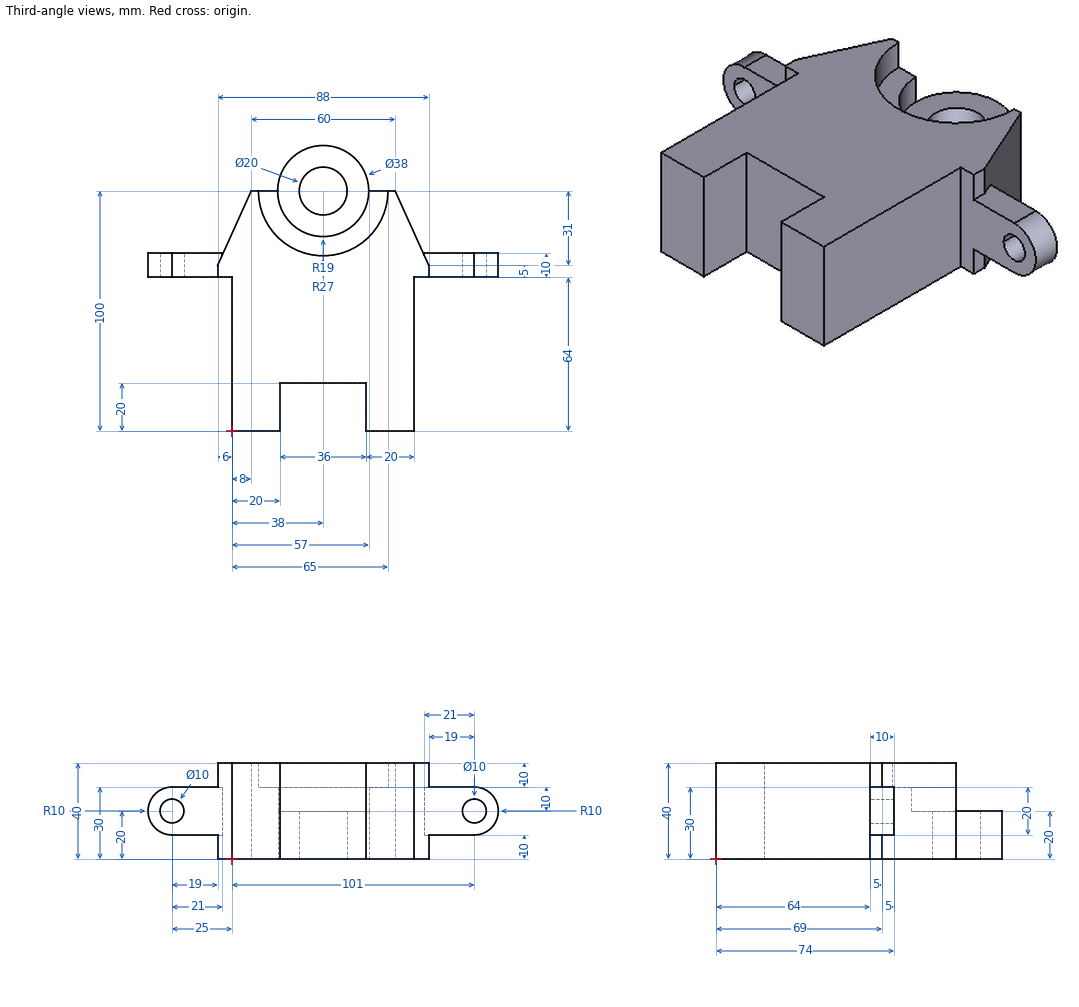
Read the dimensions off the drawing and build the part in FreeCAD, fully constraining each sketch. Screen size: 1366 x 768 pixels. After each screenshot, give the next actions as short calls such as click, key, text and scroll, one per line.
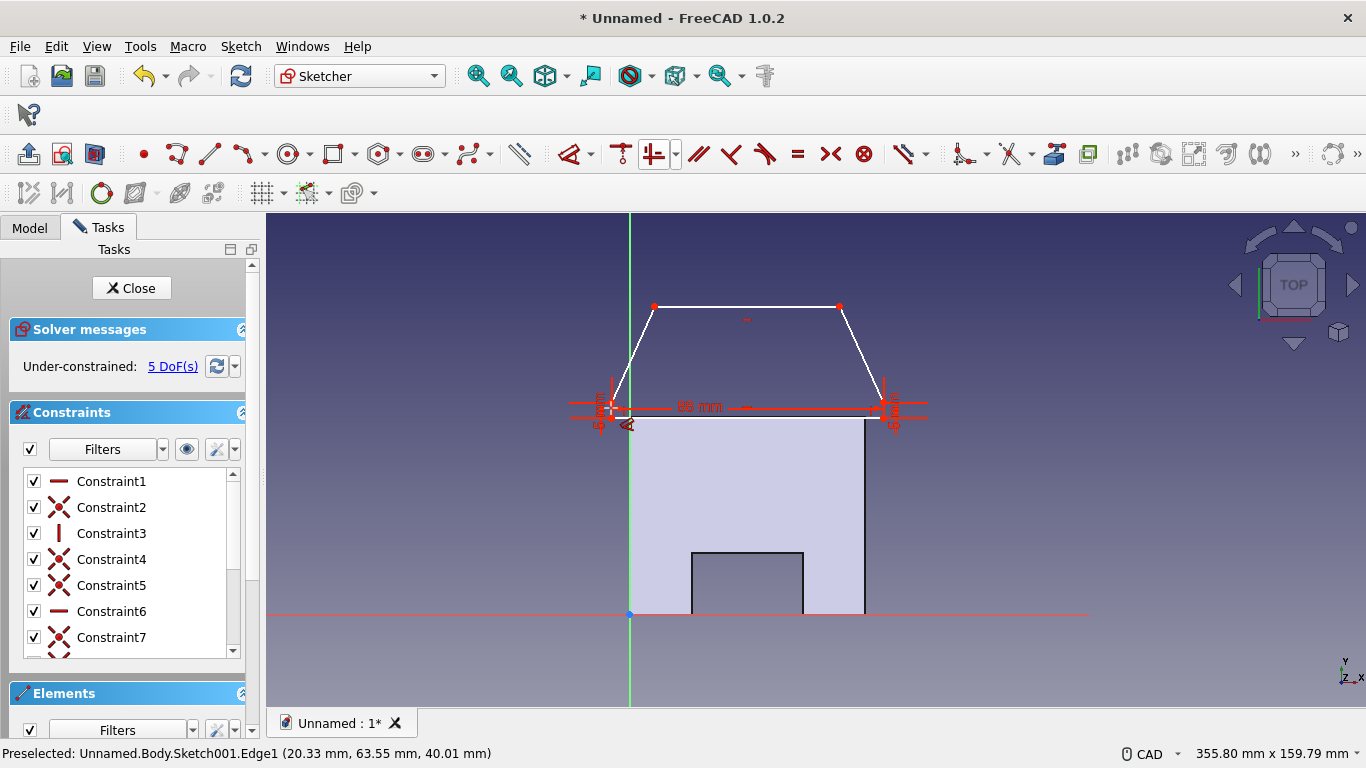
click(784, 307)
click(747, 273)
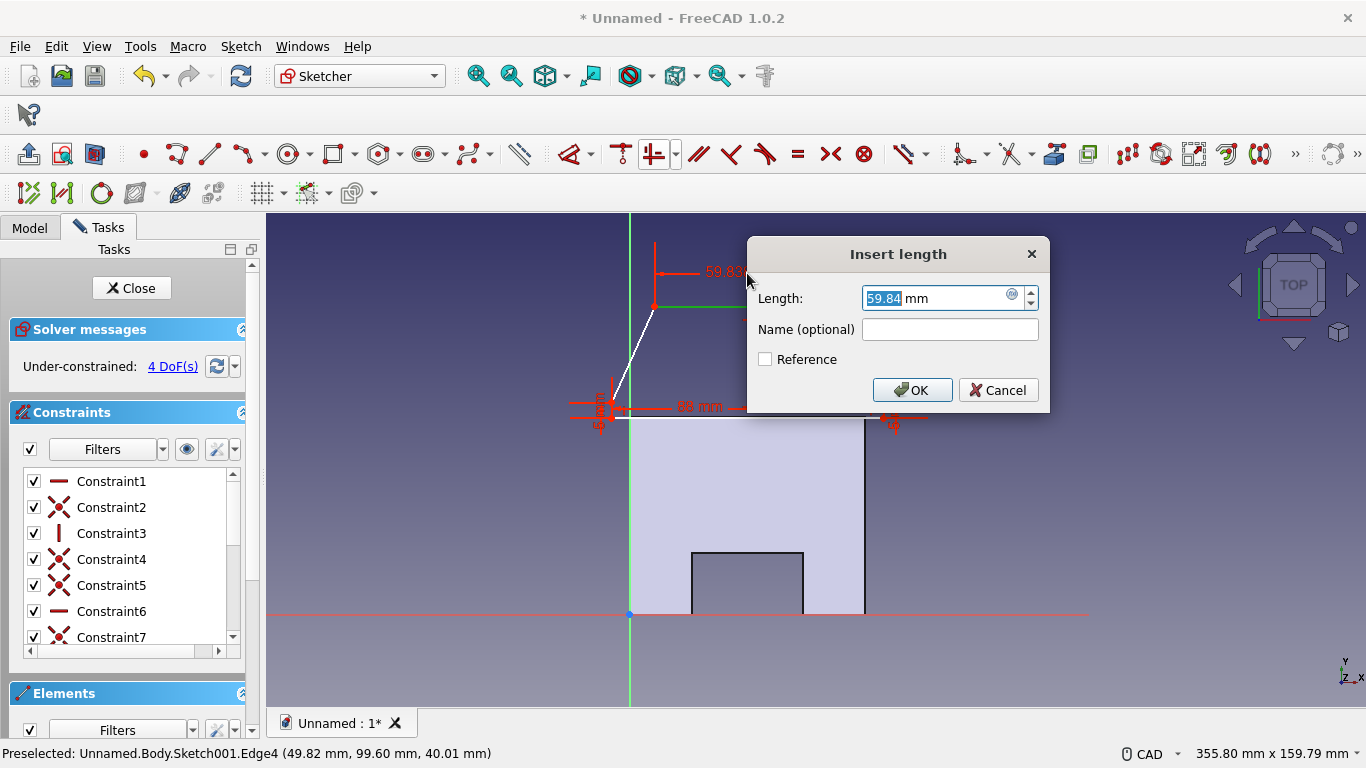
text(60)
key(Return)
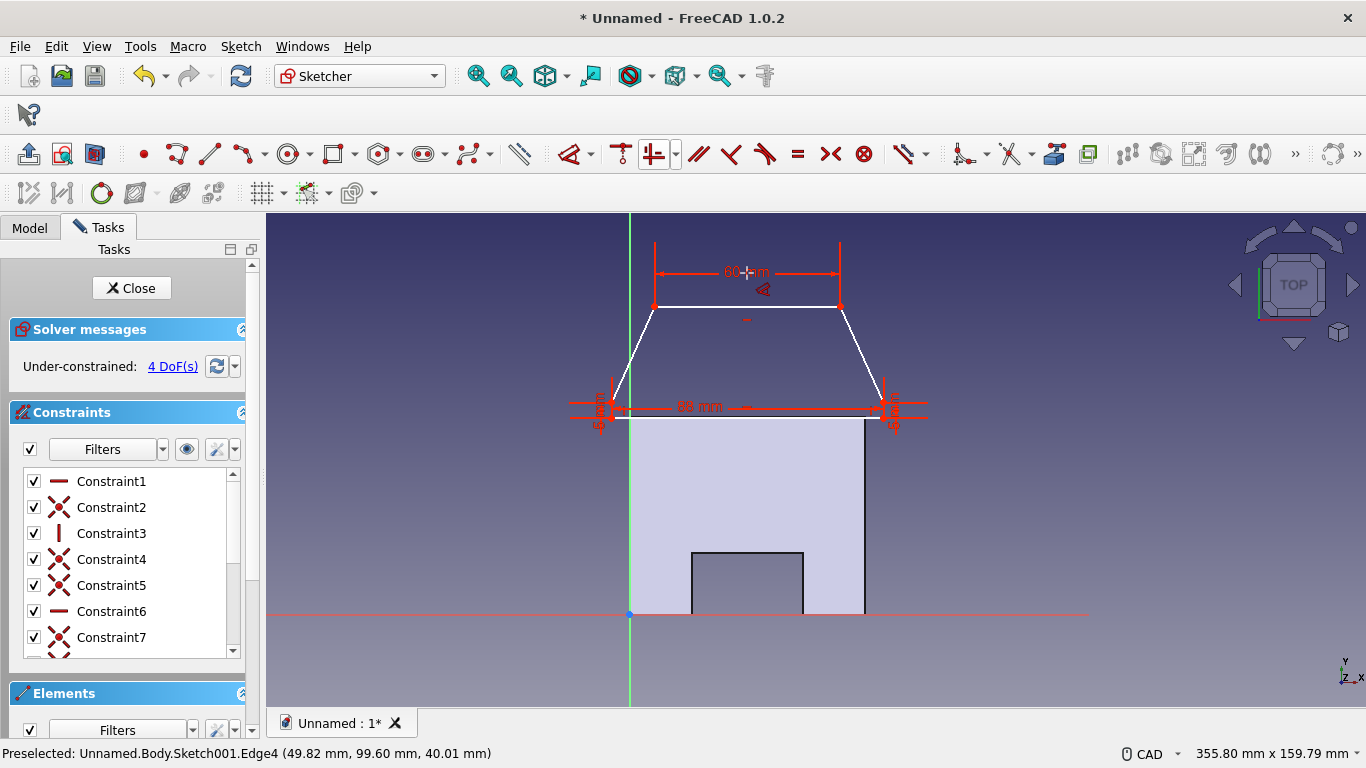
scroll(612, 418, up, 4)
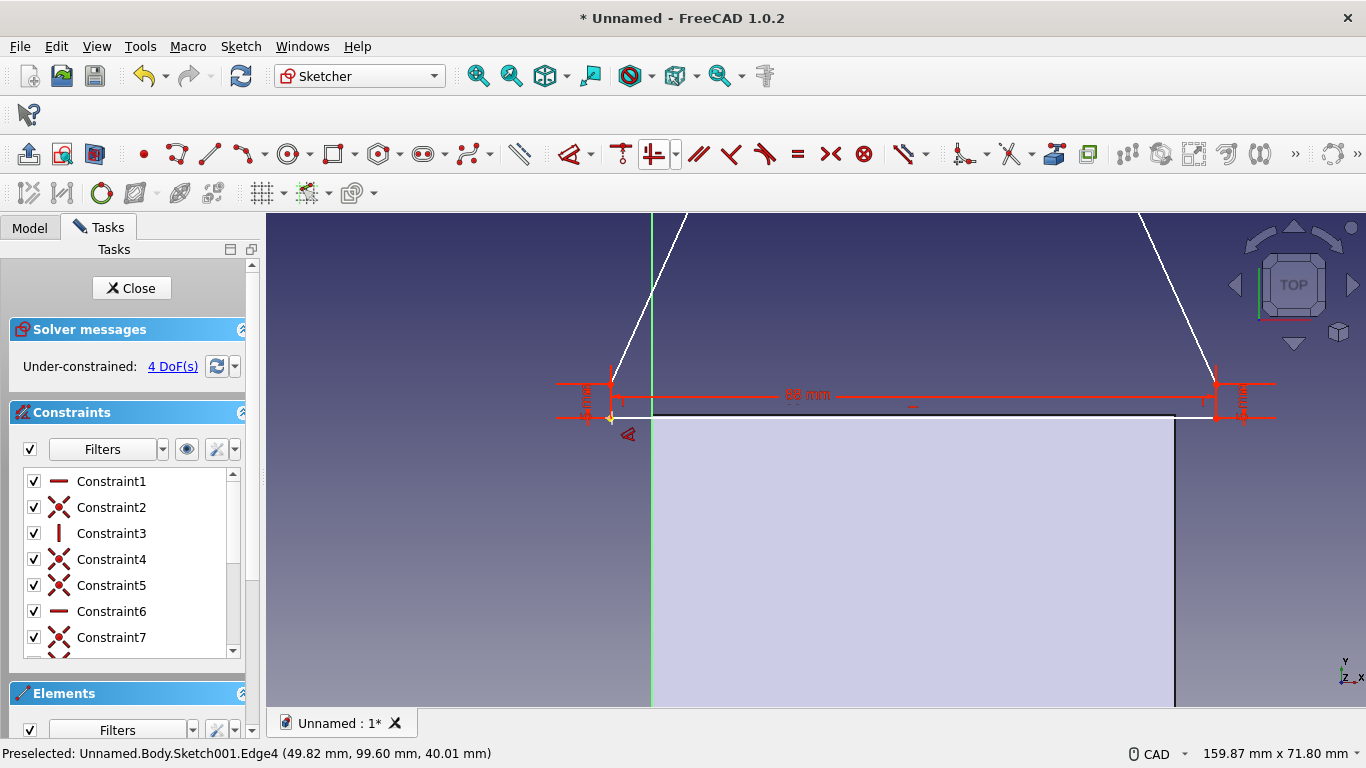
click(611, 418)
click(617, 336)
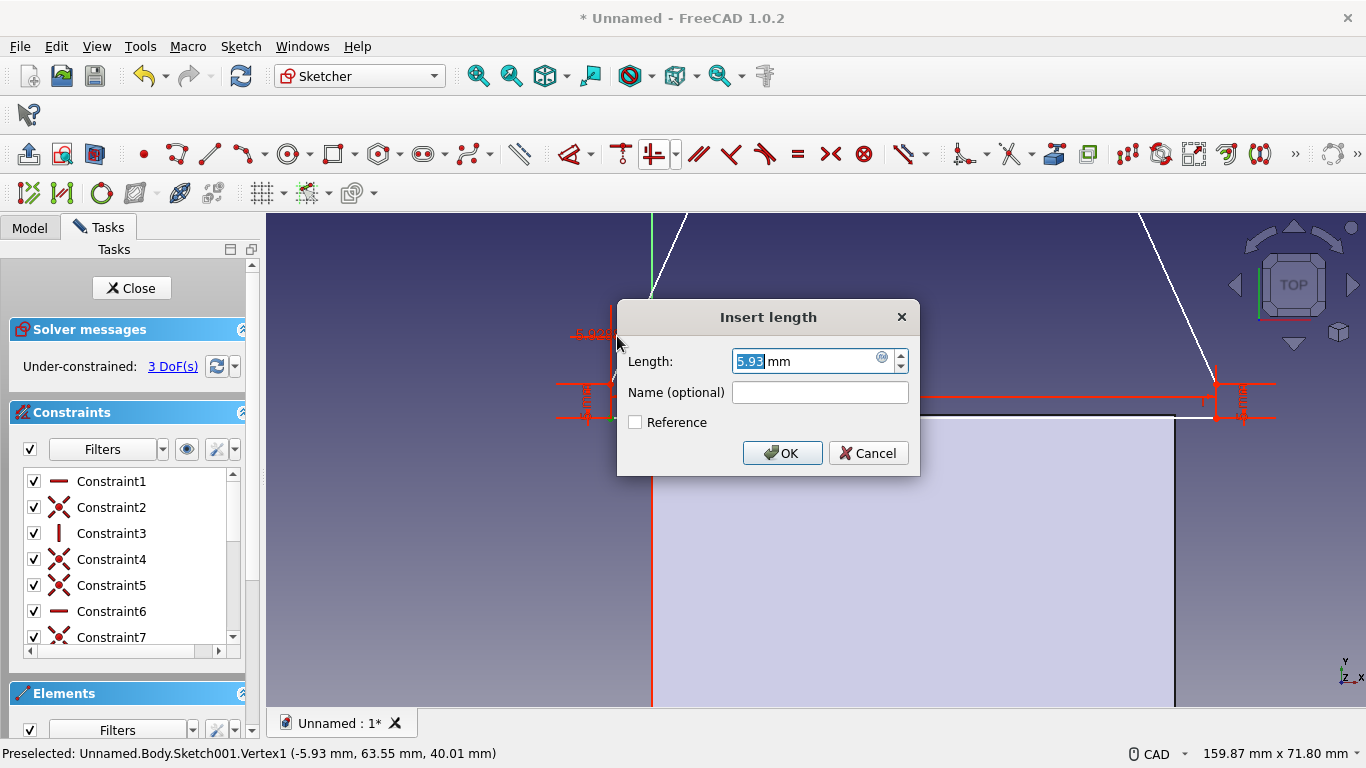
text(6)
key(Return)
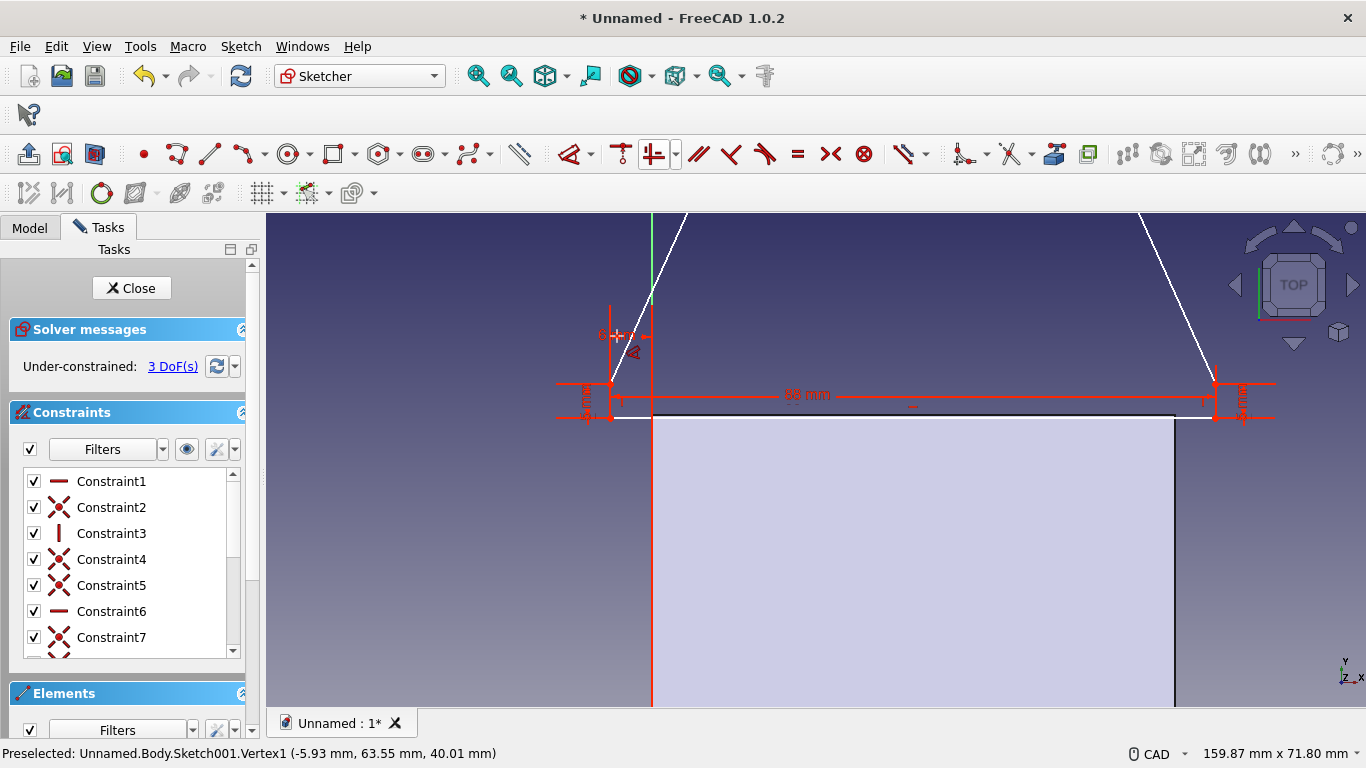
scroll(612, 418, down, 4)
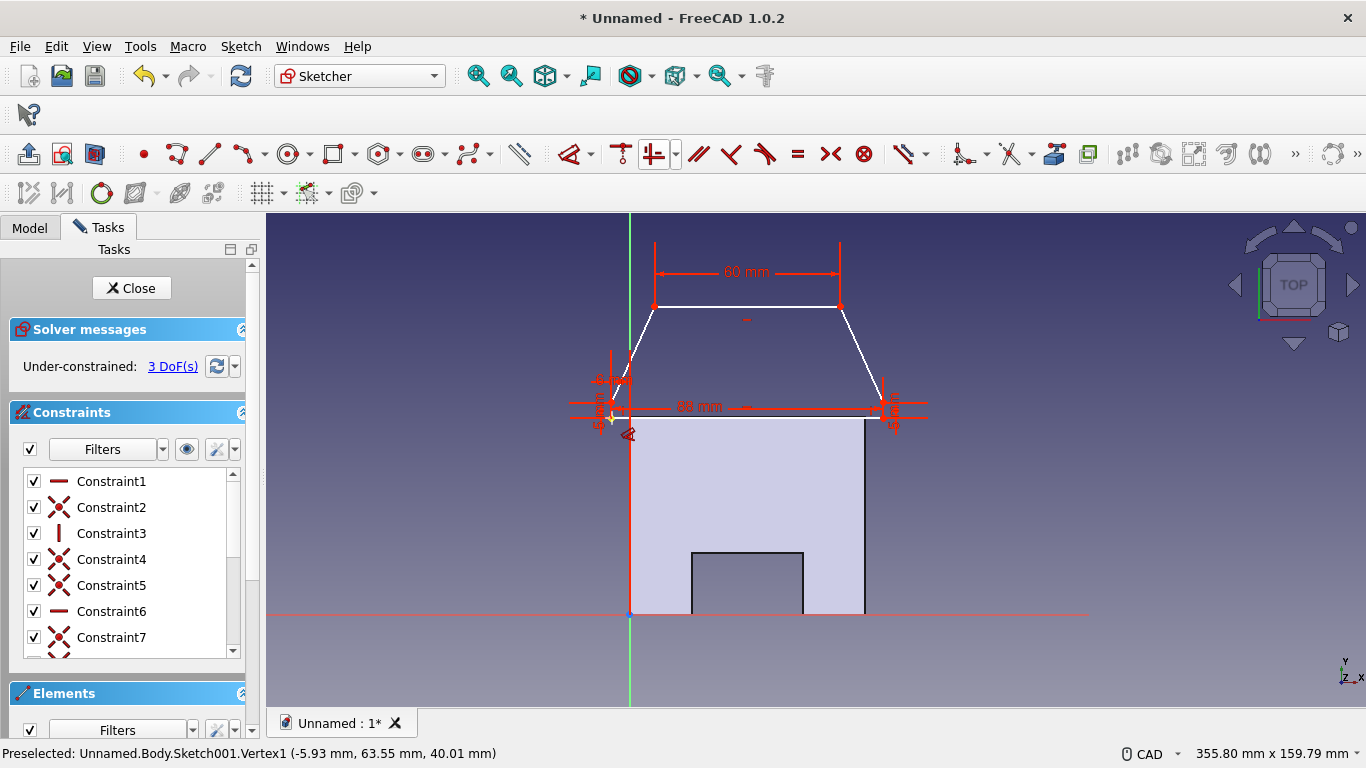
scroll(655, 307, up, 3)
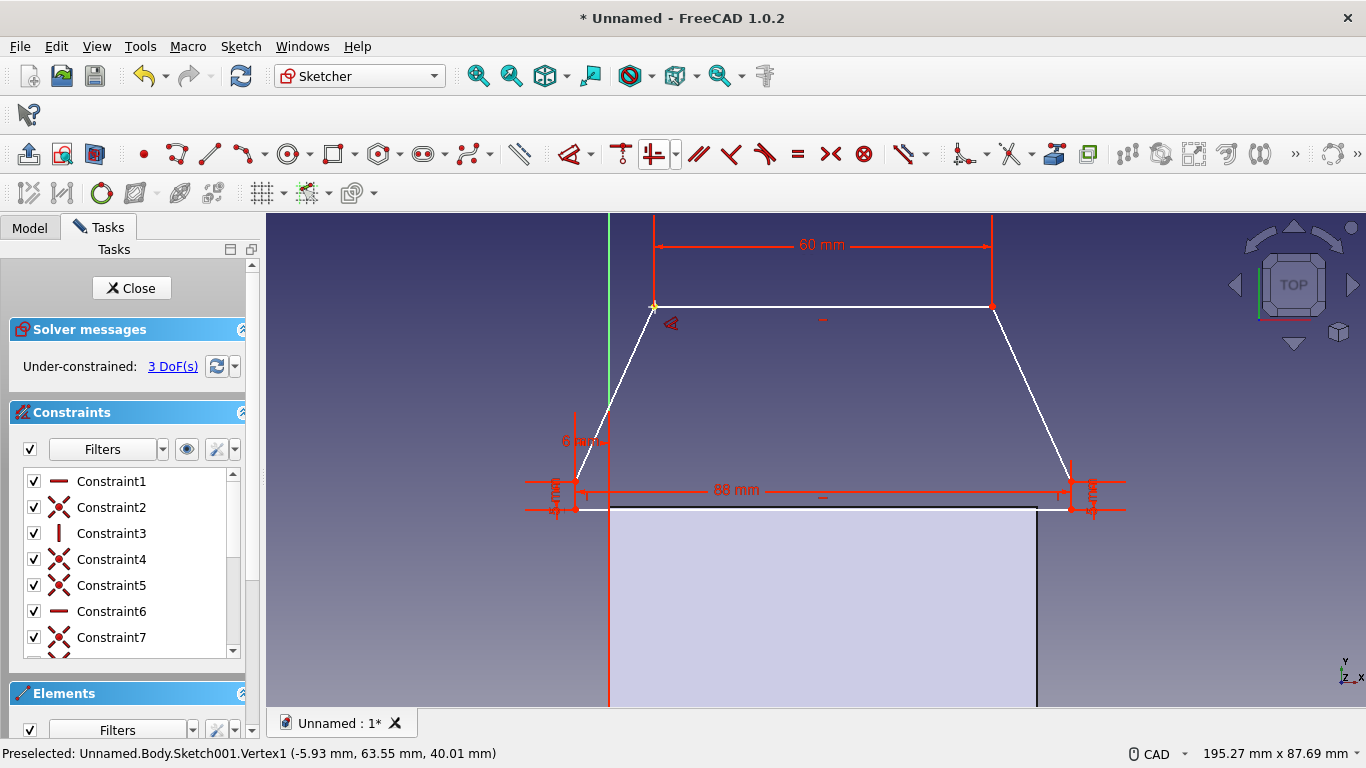
click(654, 307)
click(632, 273)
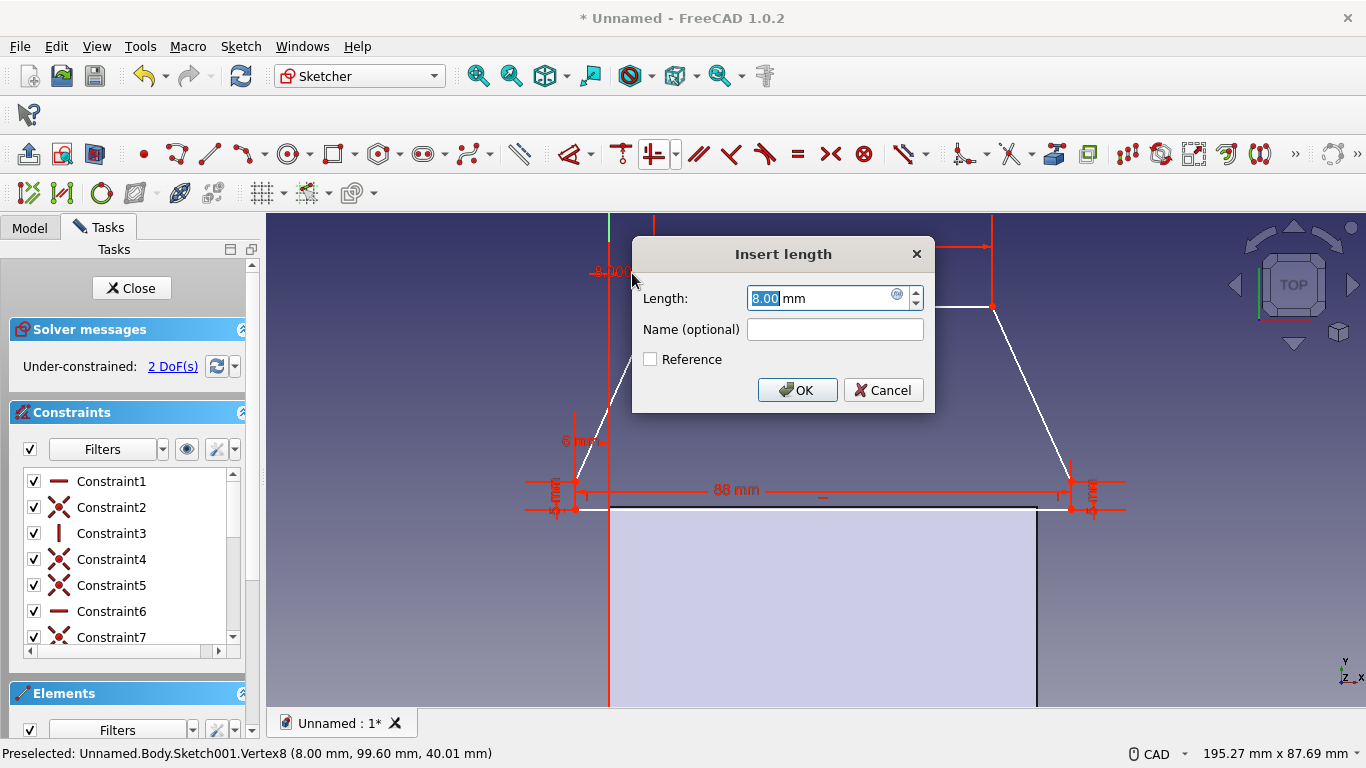
text(8)
key(Return)